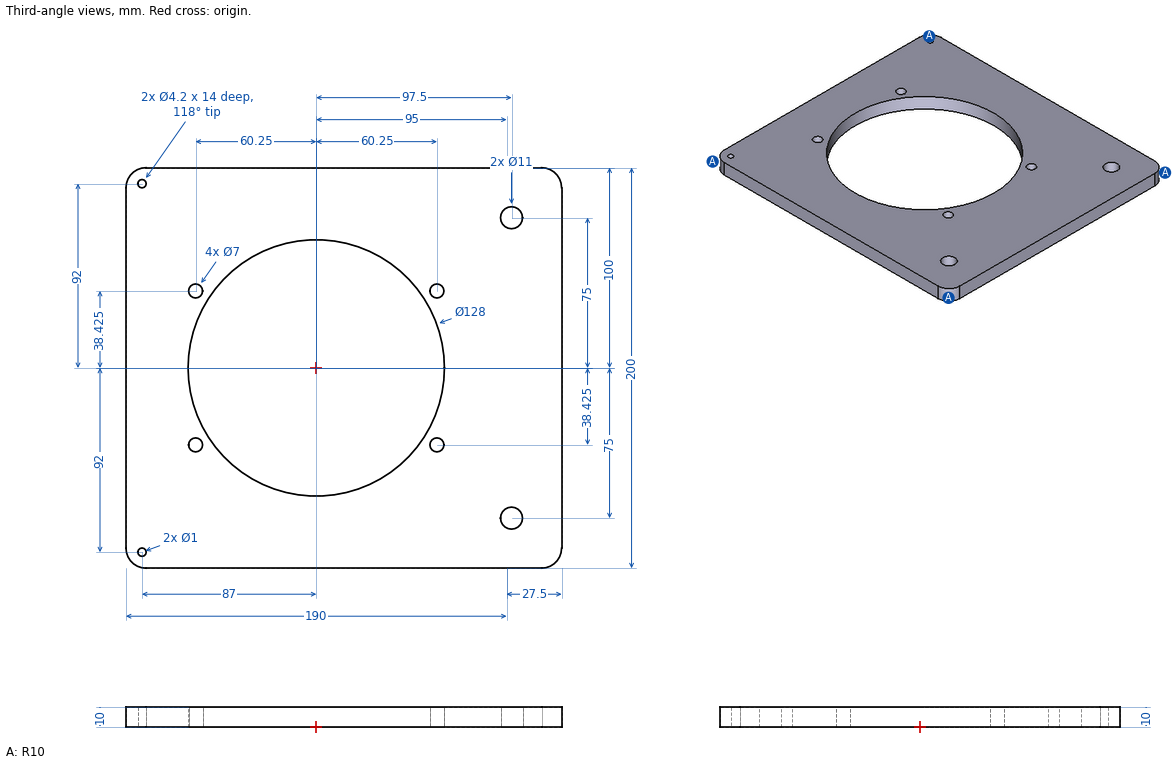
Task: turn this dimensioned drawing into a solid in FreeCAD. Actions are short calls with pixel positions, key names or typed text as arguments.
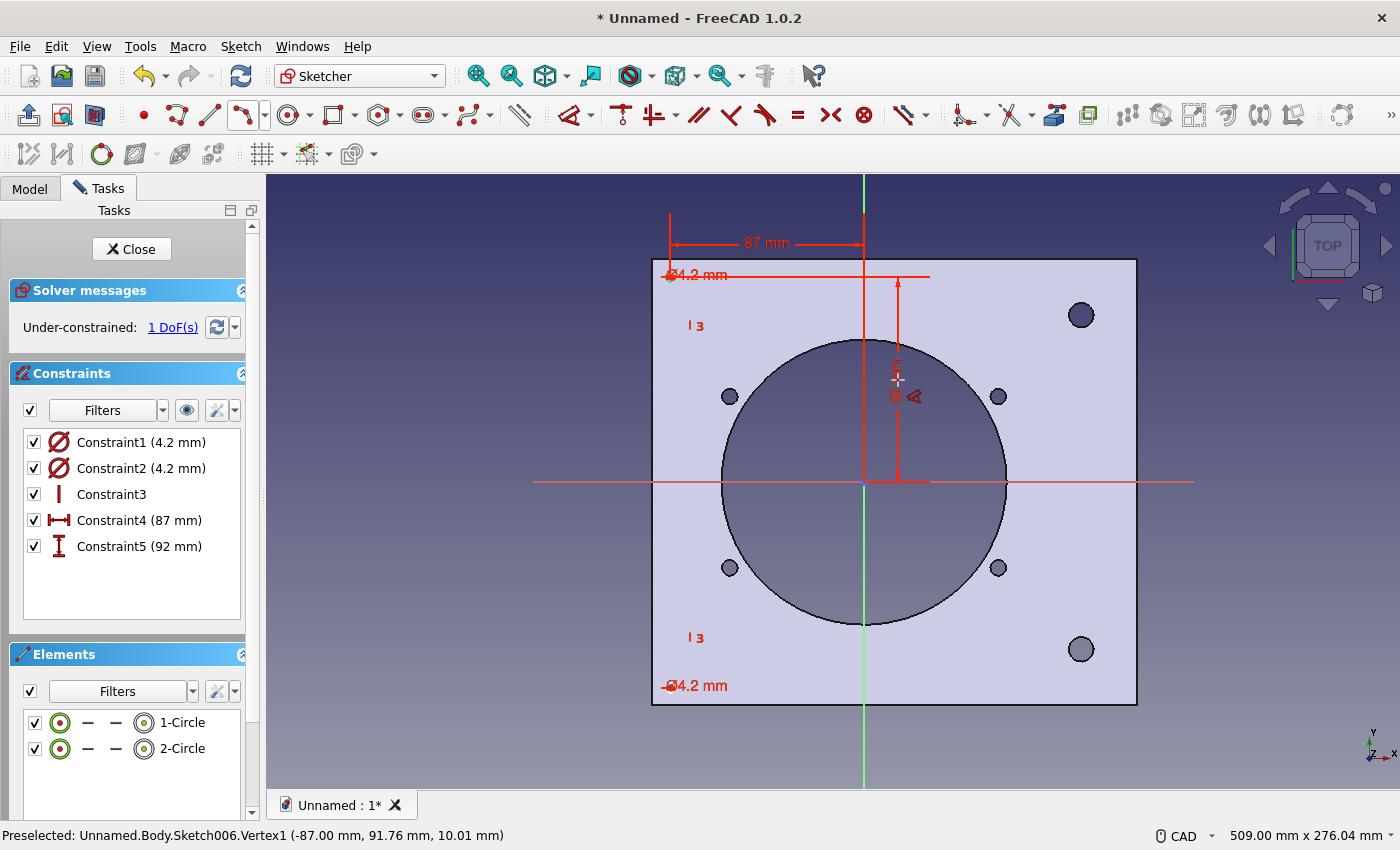
click(670, 688)
click(898, 585)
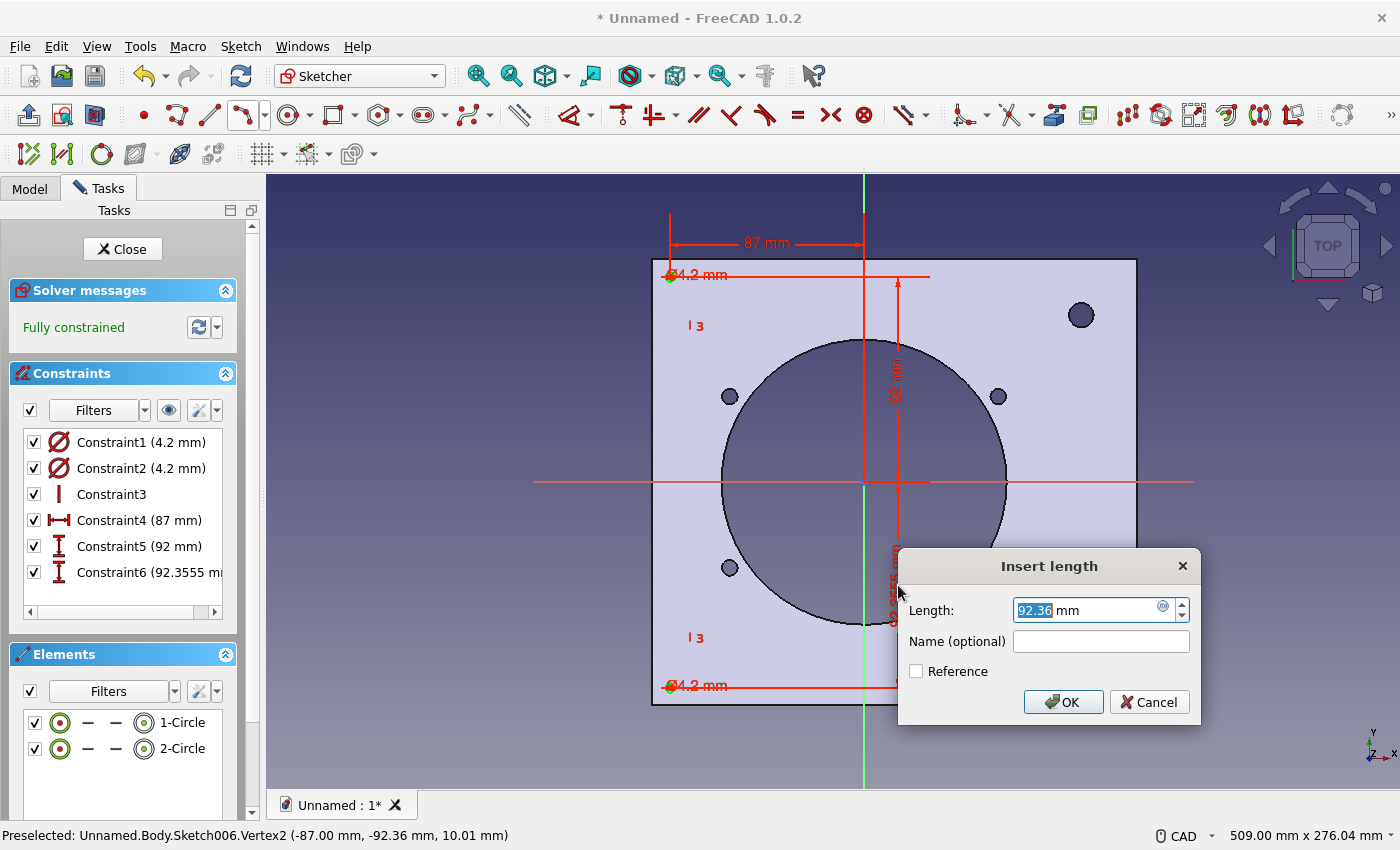
text(92)
key(Return)
key(Escape)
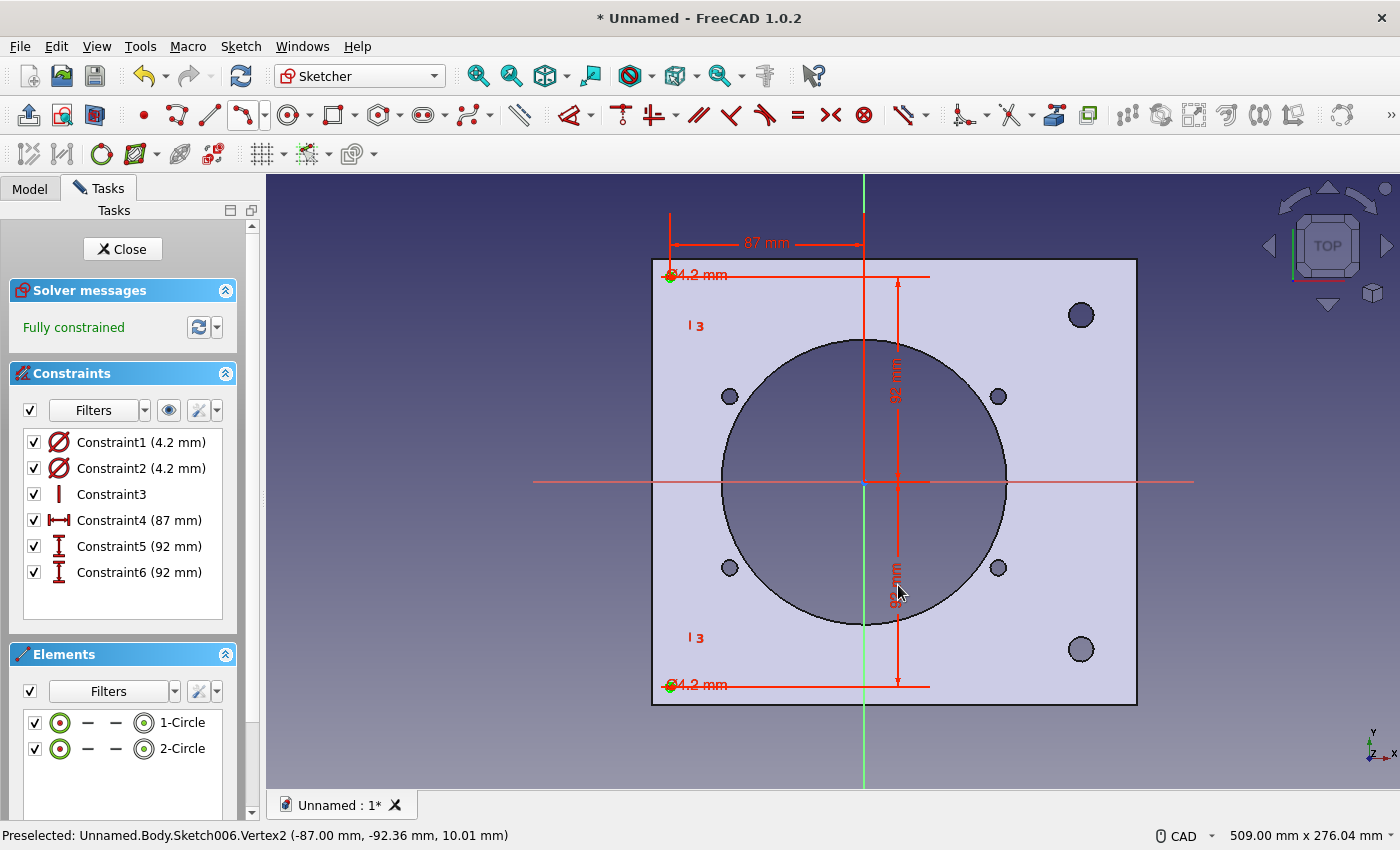
click(123, 249)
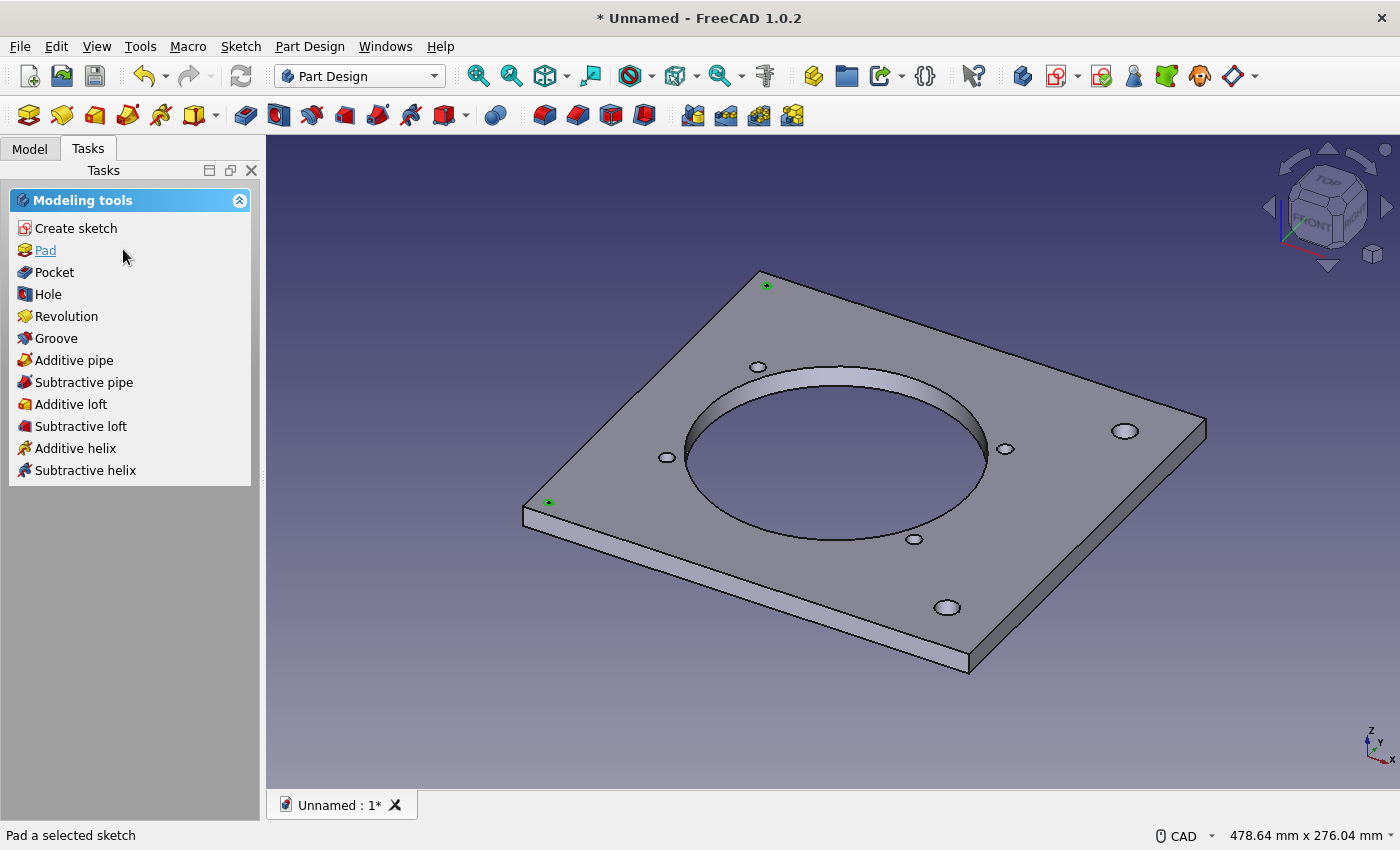
click(279, 116)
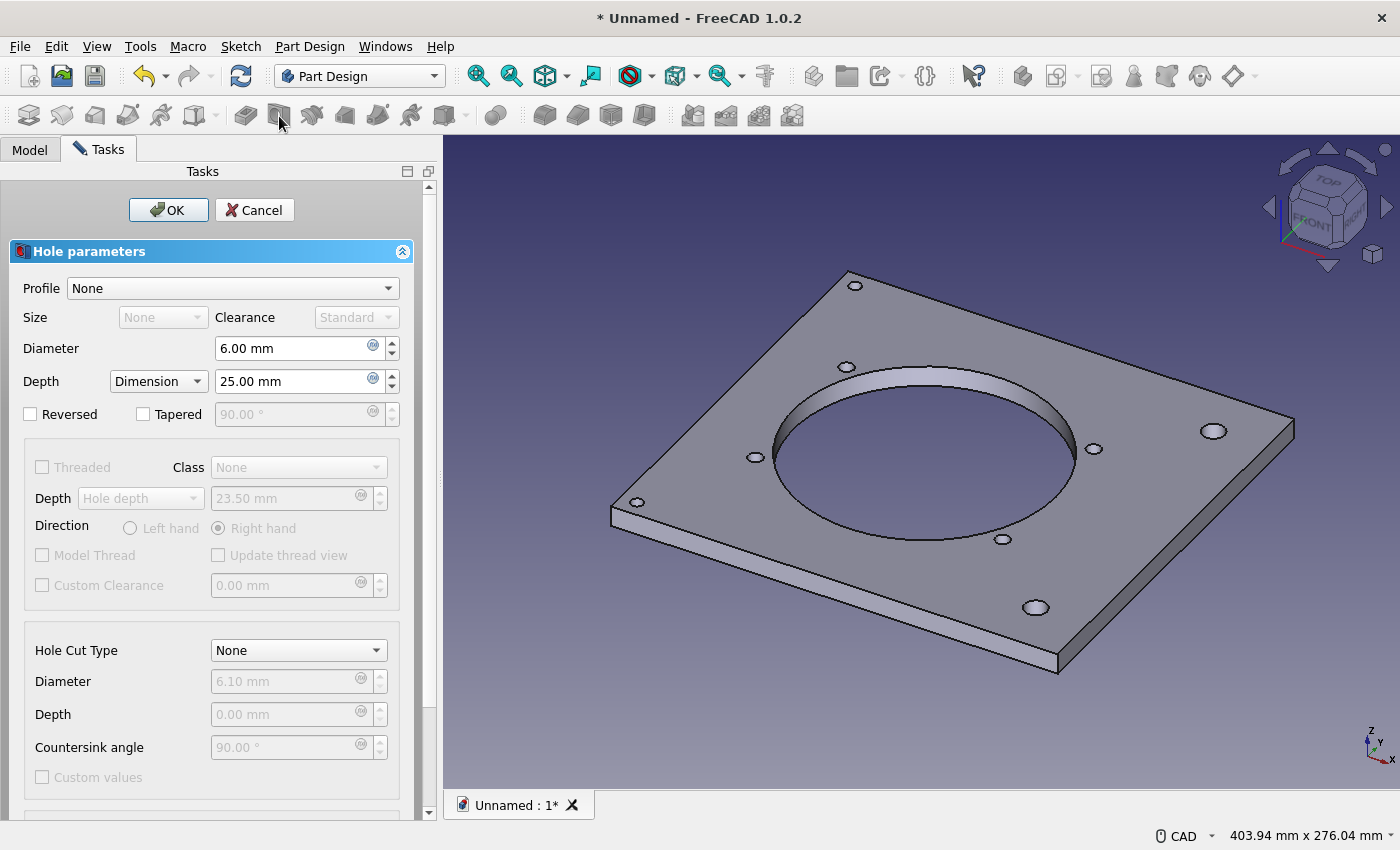
triple_click(300, 348)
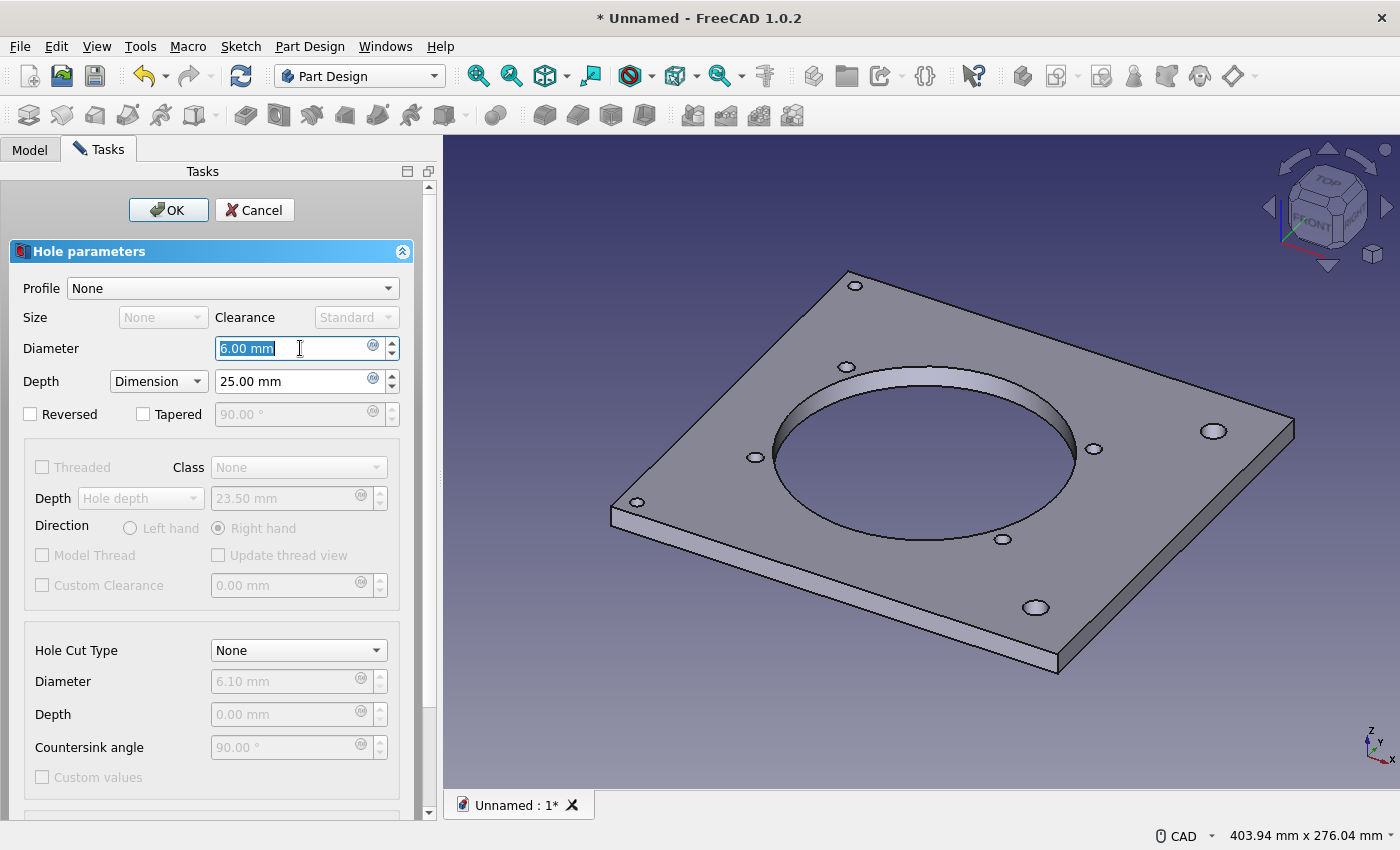
text(4.2)
key(Tab)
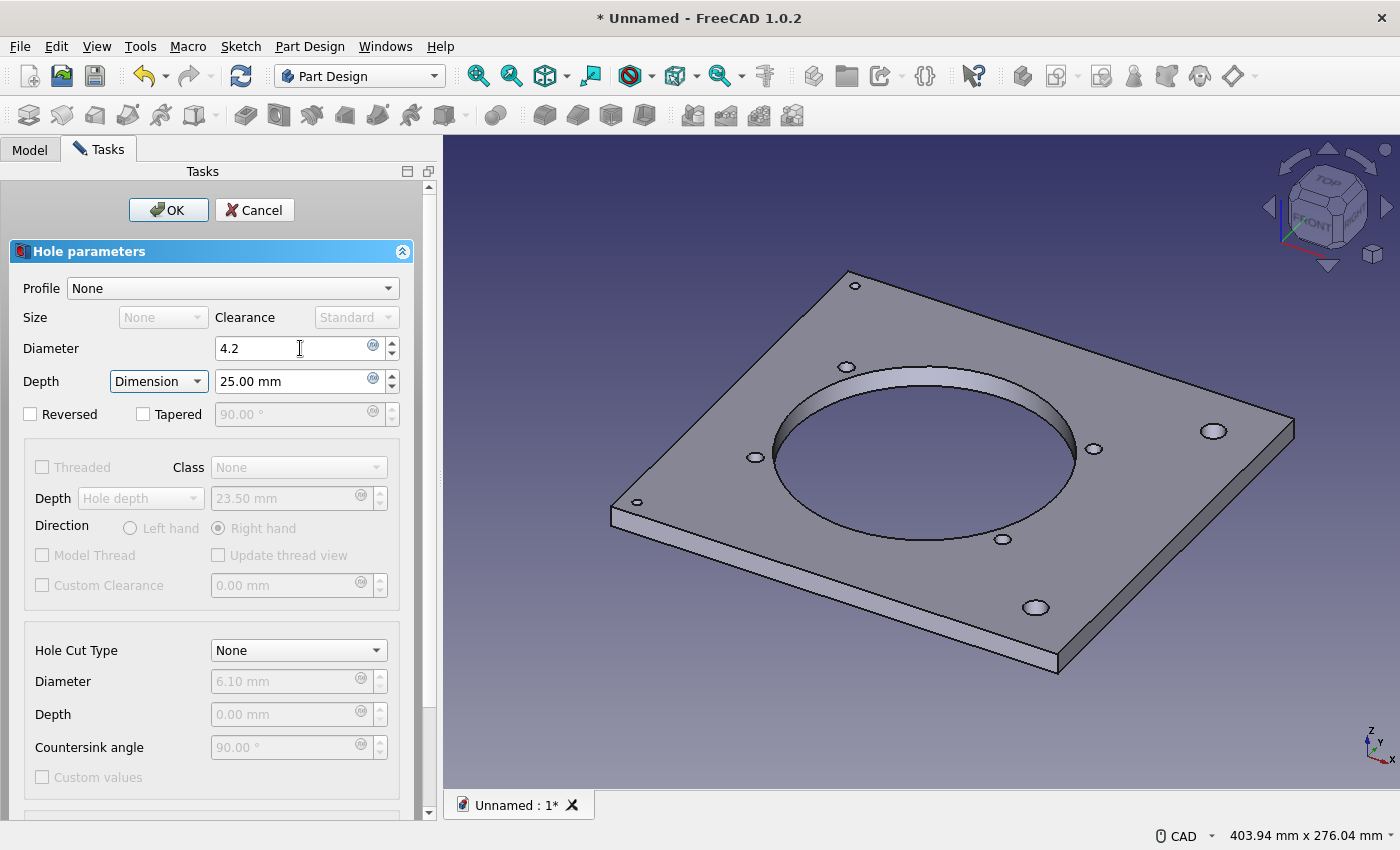
triple_click(300, 382)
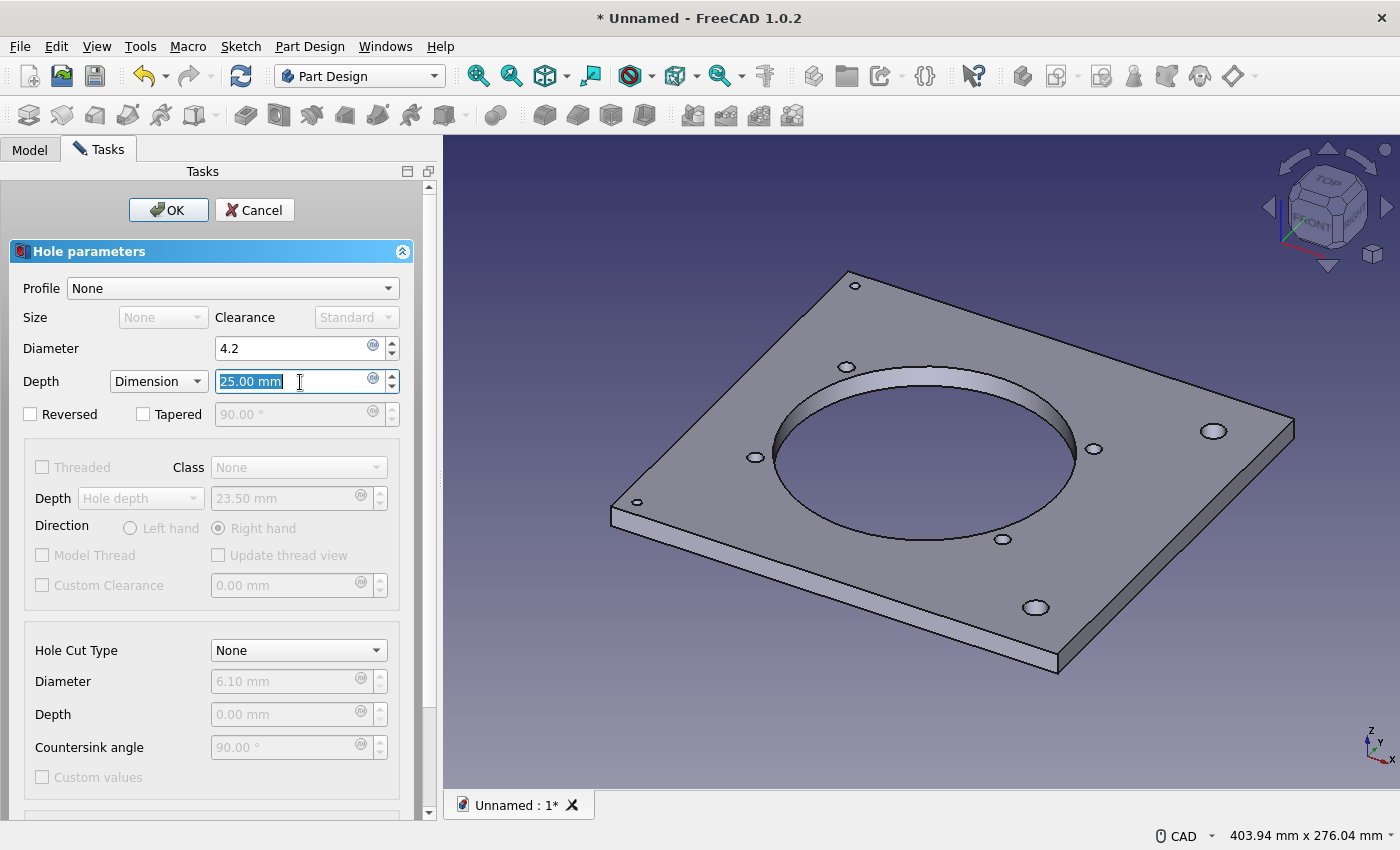
text(14)
key(Tab)